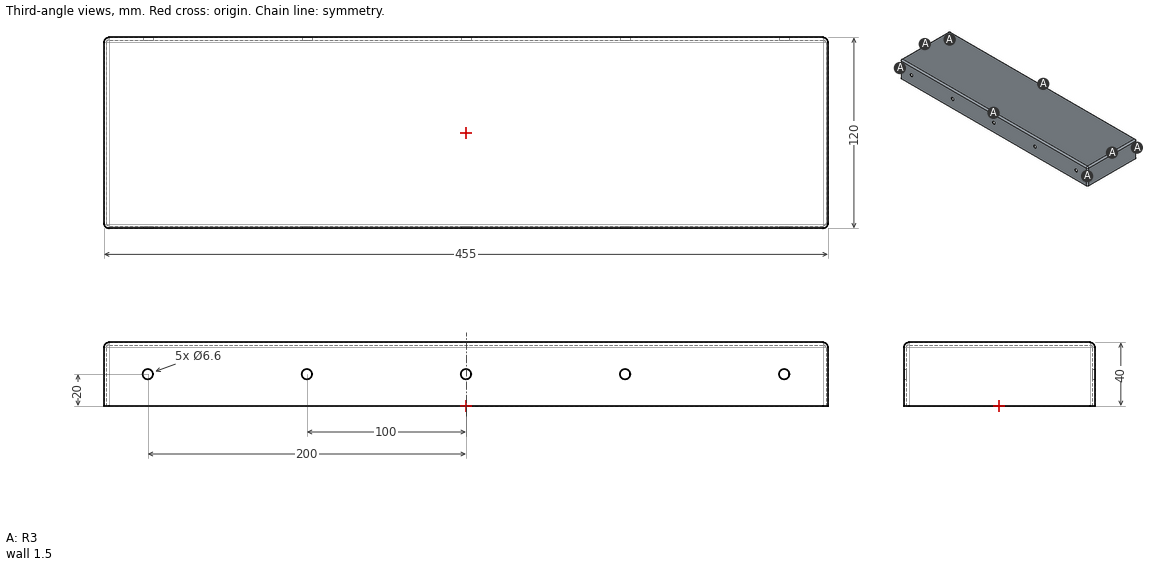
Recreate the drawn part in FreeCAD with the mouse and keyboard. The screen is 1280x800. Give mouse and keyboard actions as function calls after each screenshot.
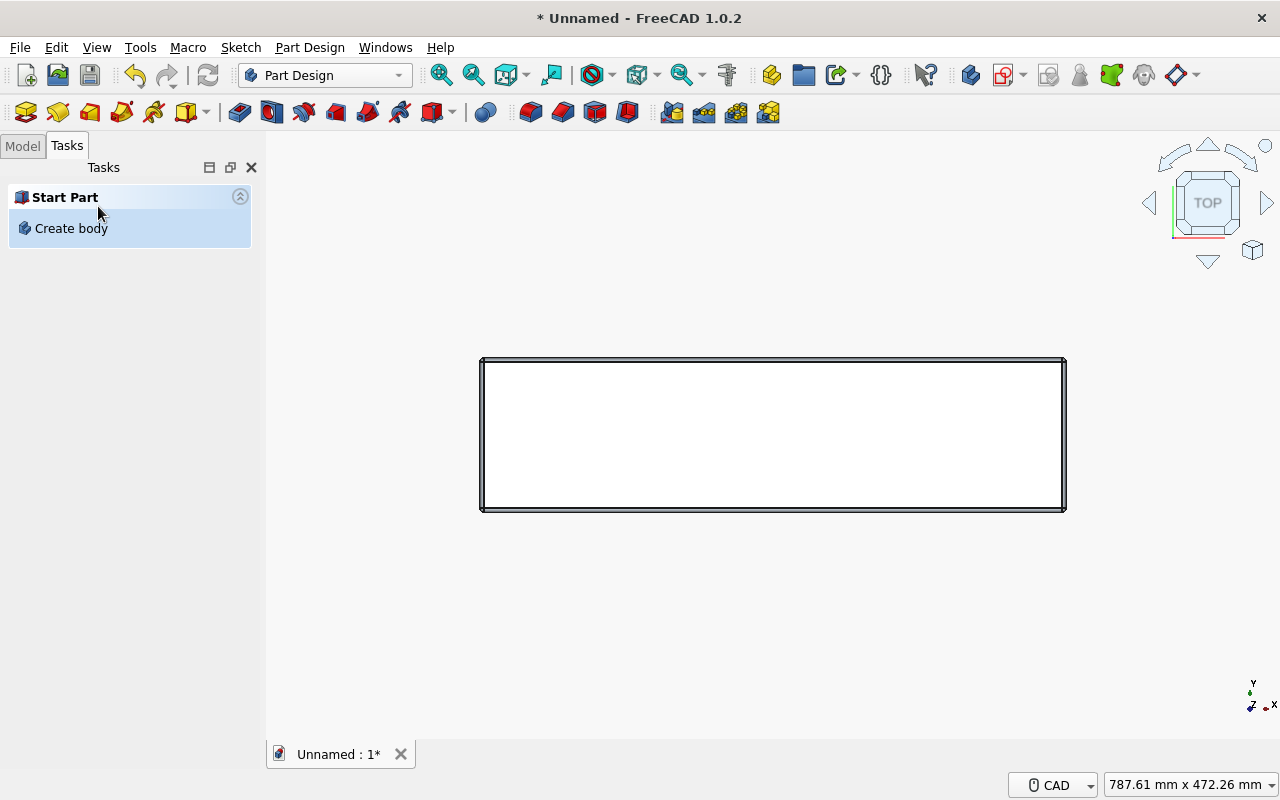
key(1)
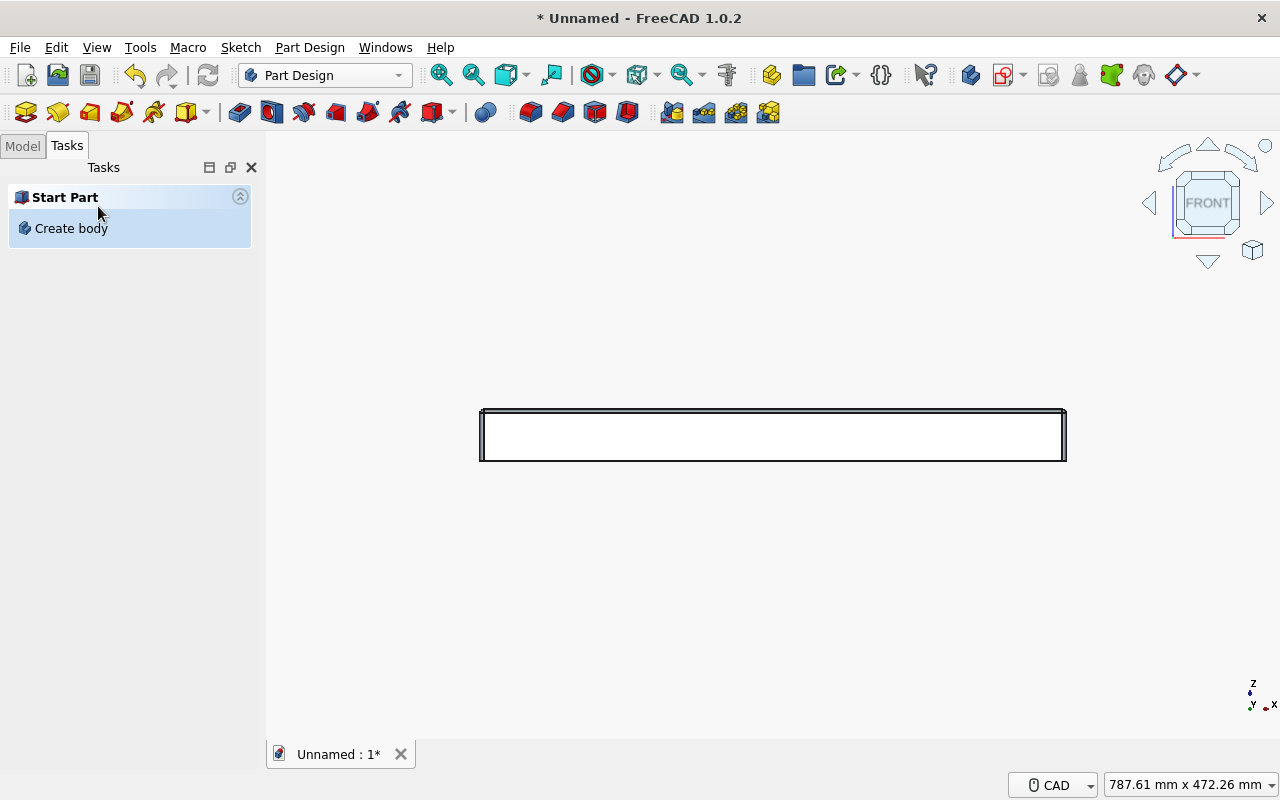
key(3)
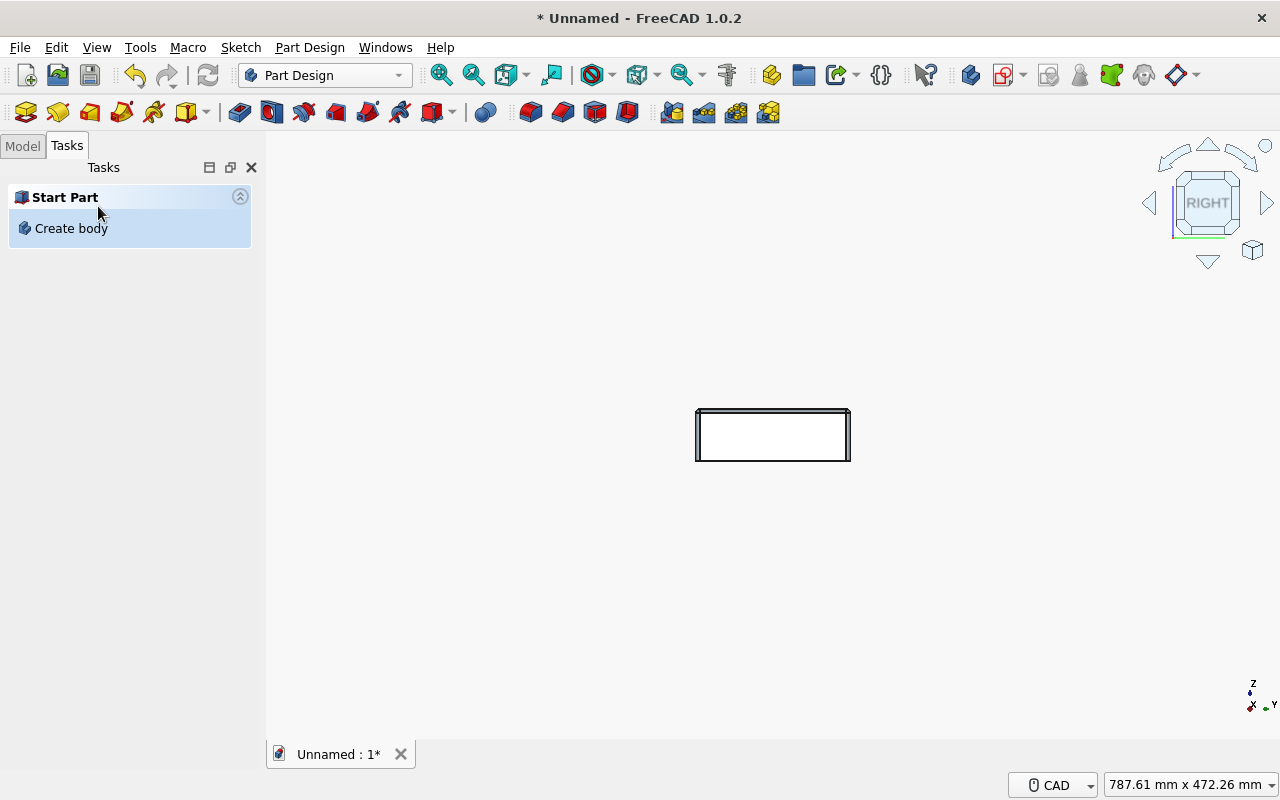
click(442, 76)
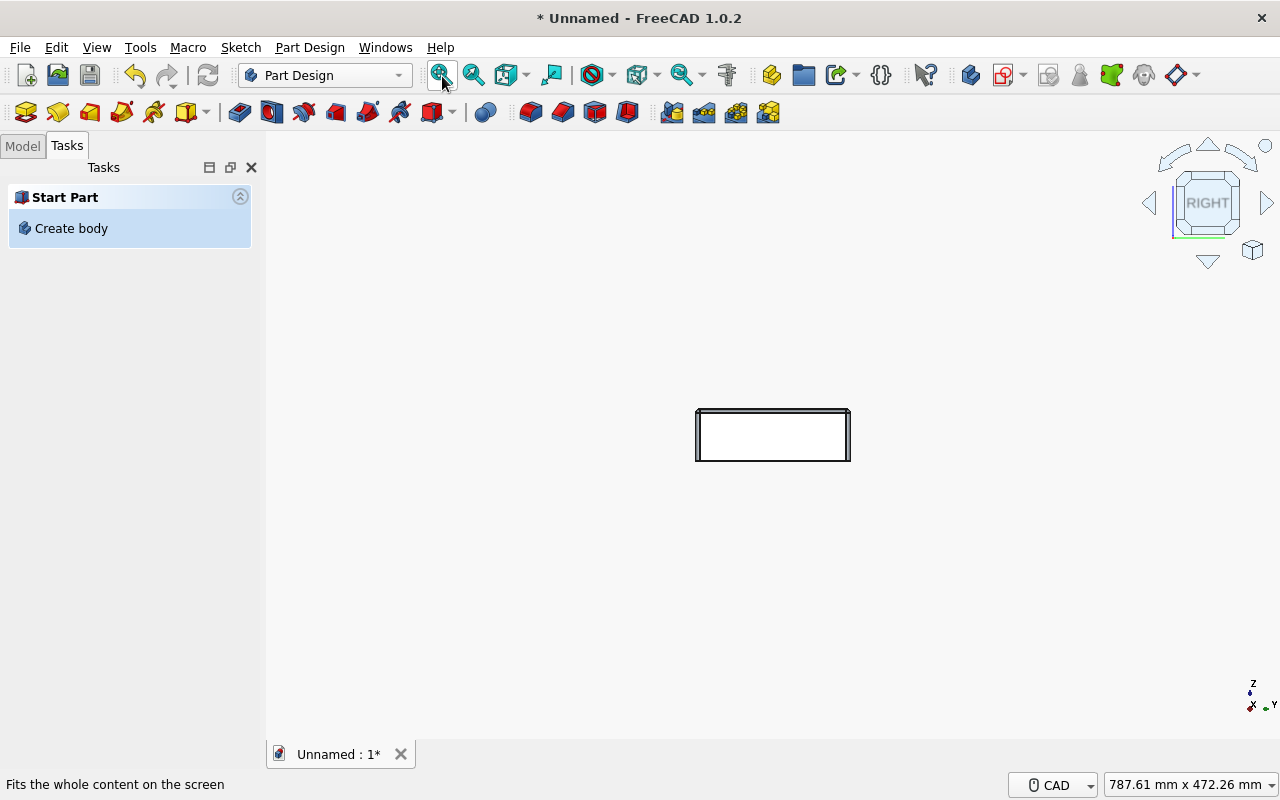
key(5)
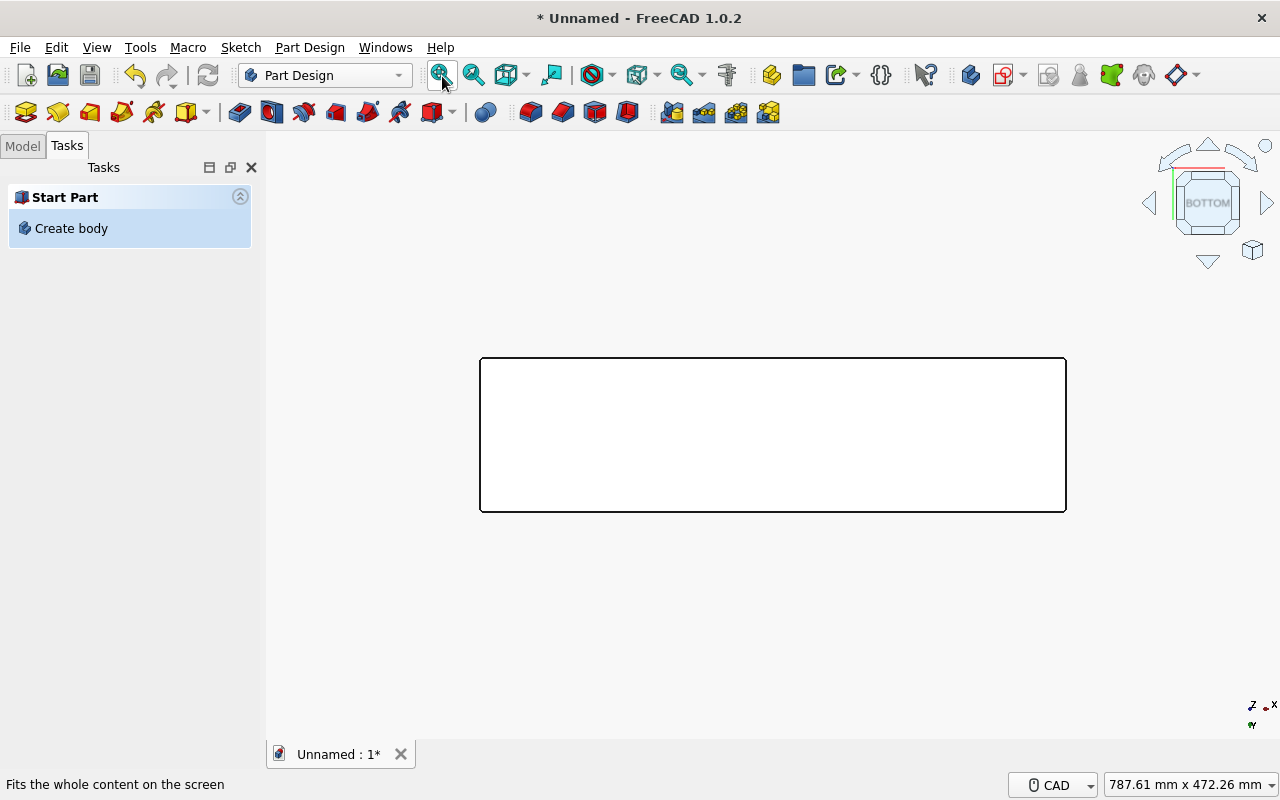
click(940, 434)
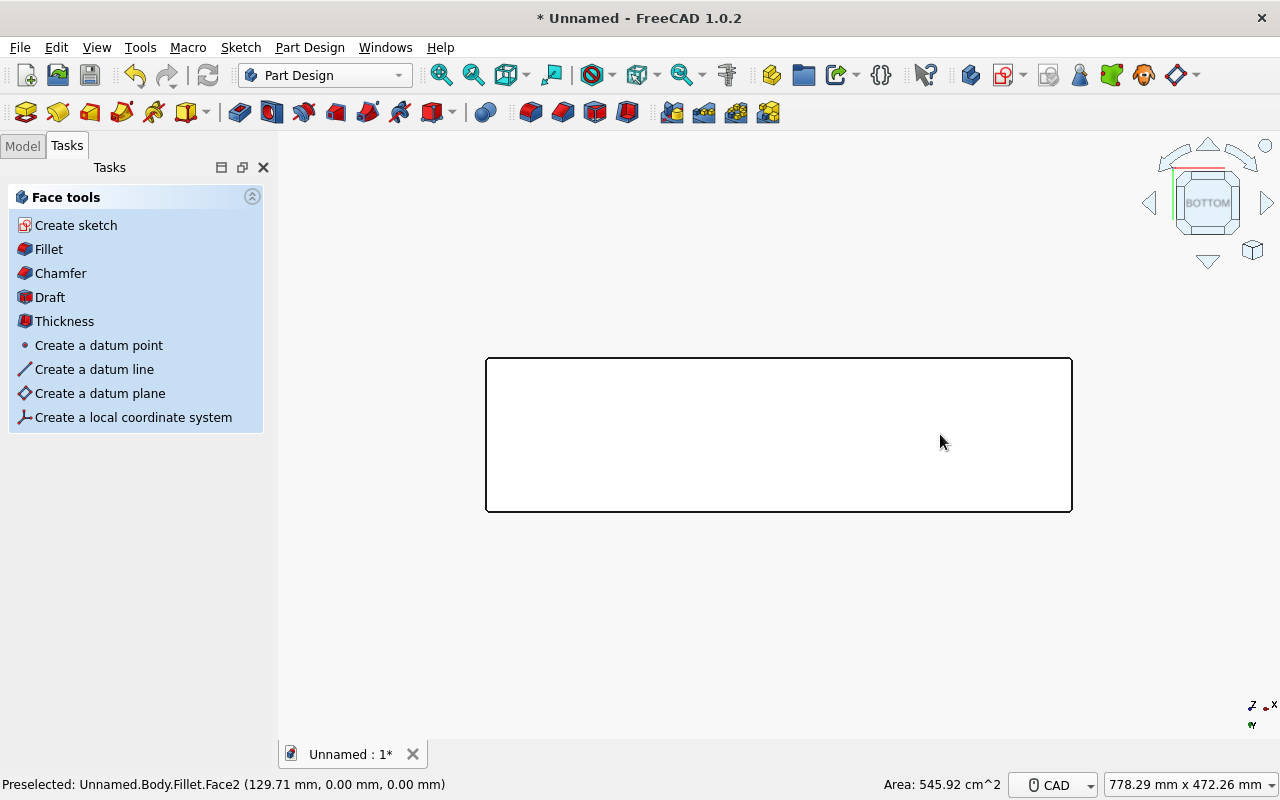
click(628, 112)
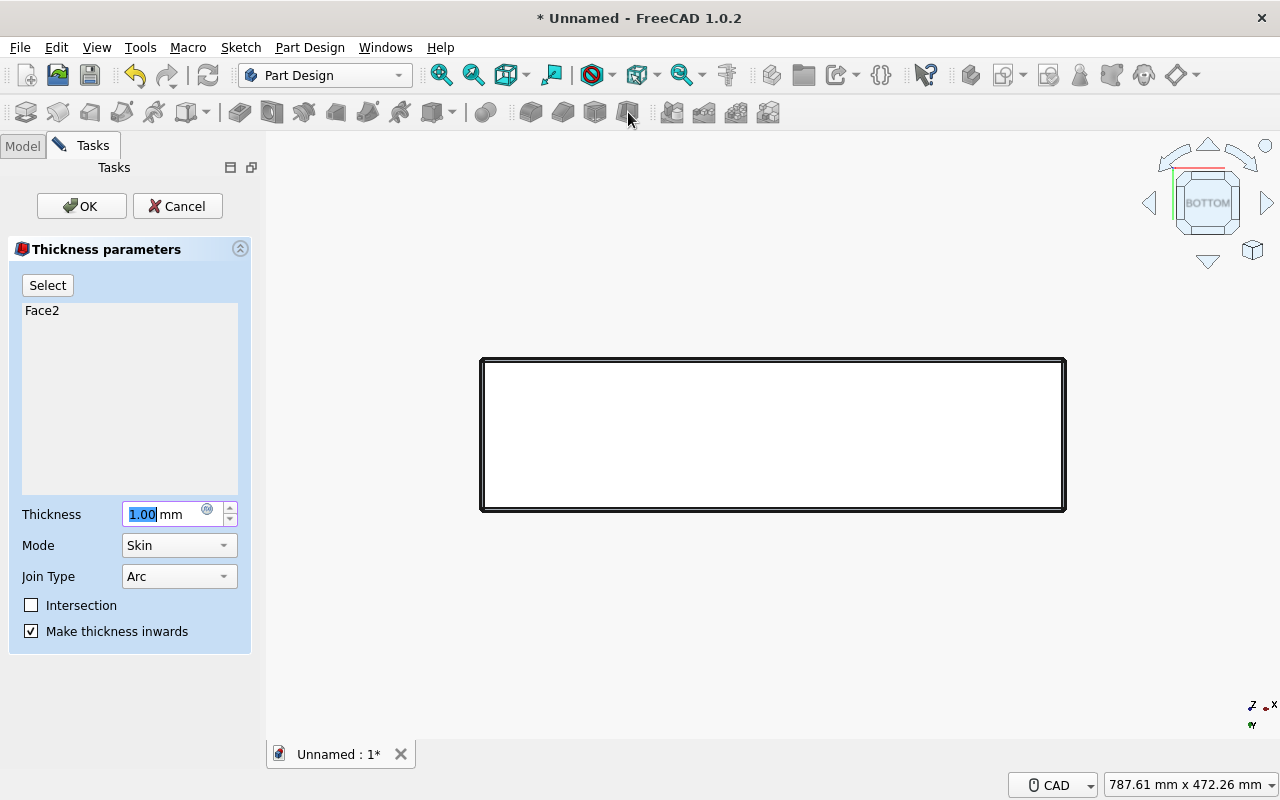
text(1.5)
key(Tab)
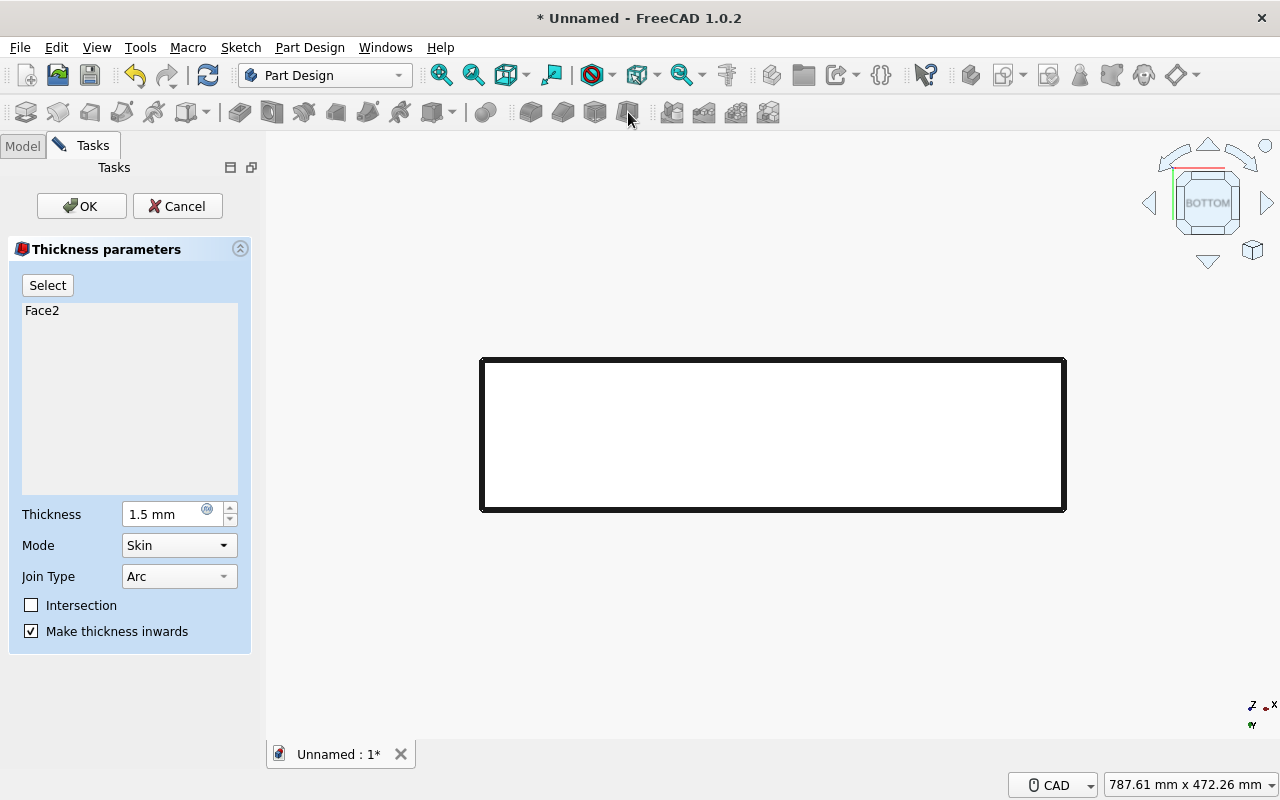
click(180, 576)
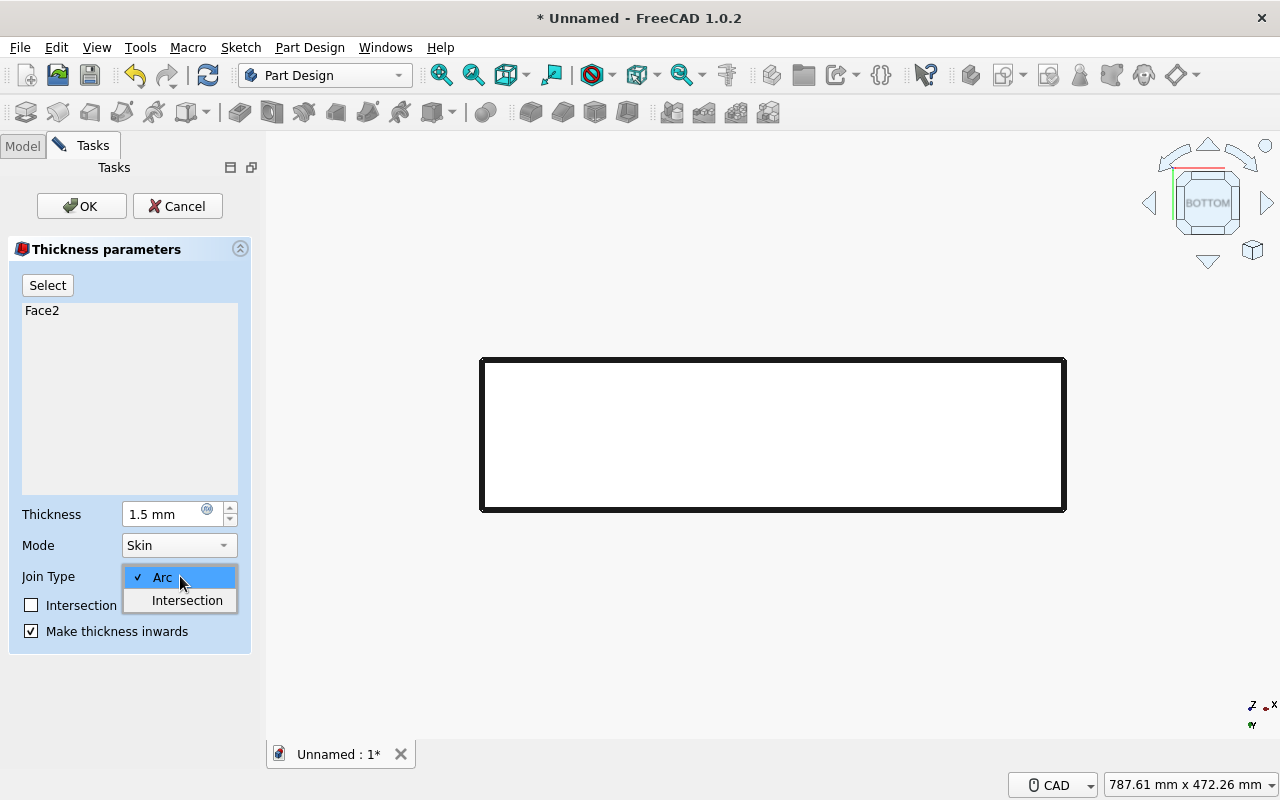
click(179, 600)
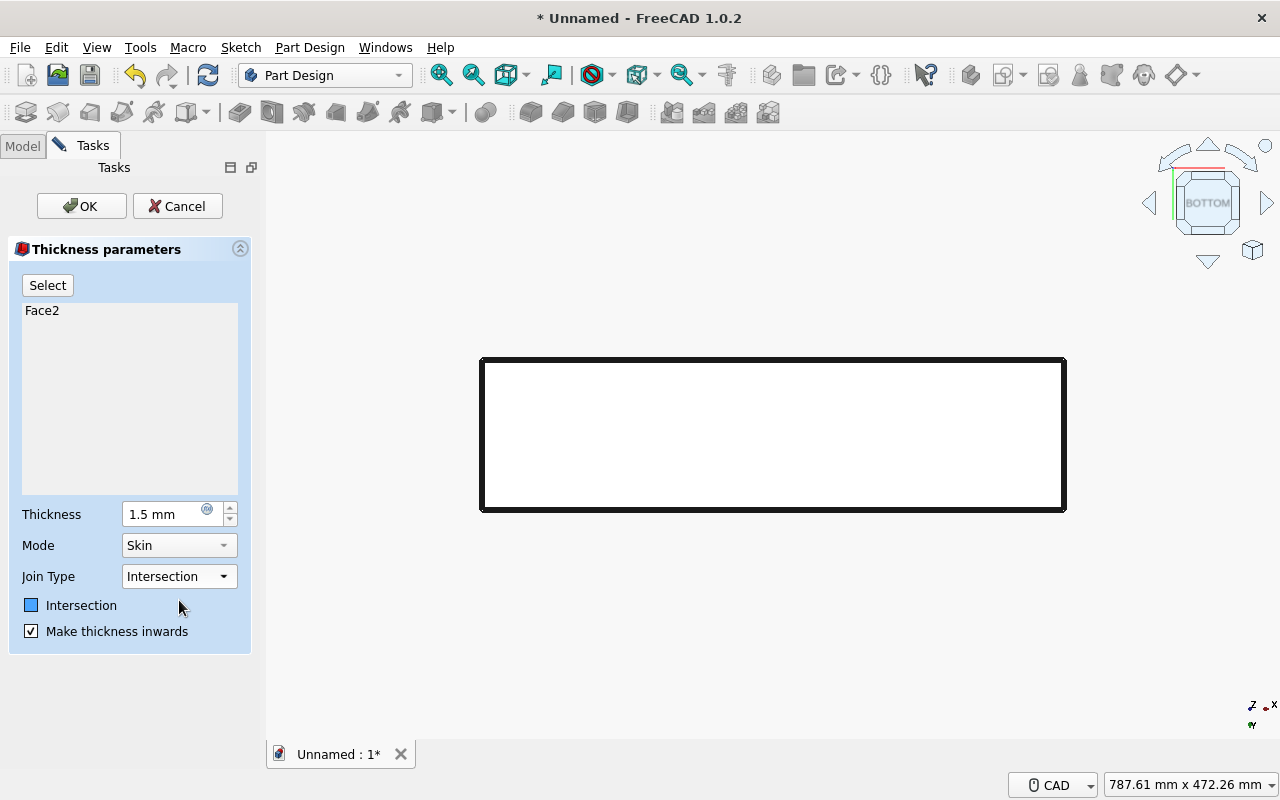
click(82, 206)